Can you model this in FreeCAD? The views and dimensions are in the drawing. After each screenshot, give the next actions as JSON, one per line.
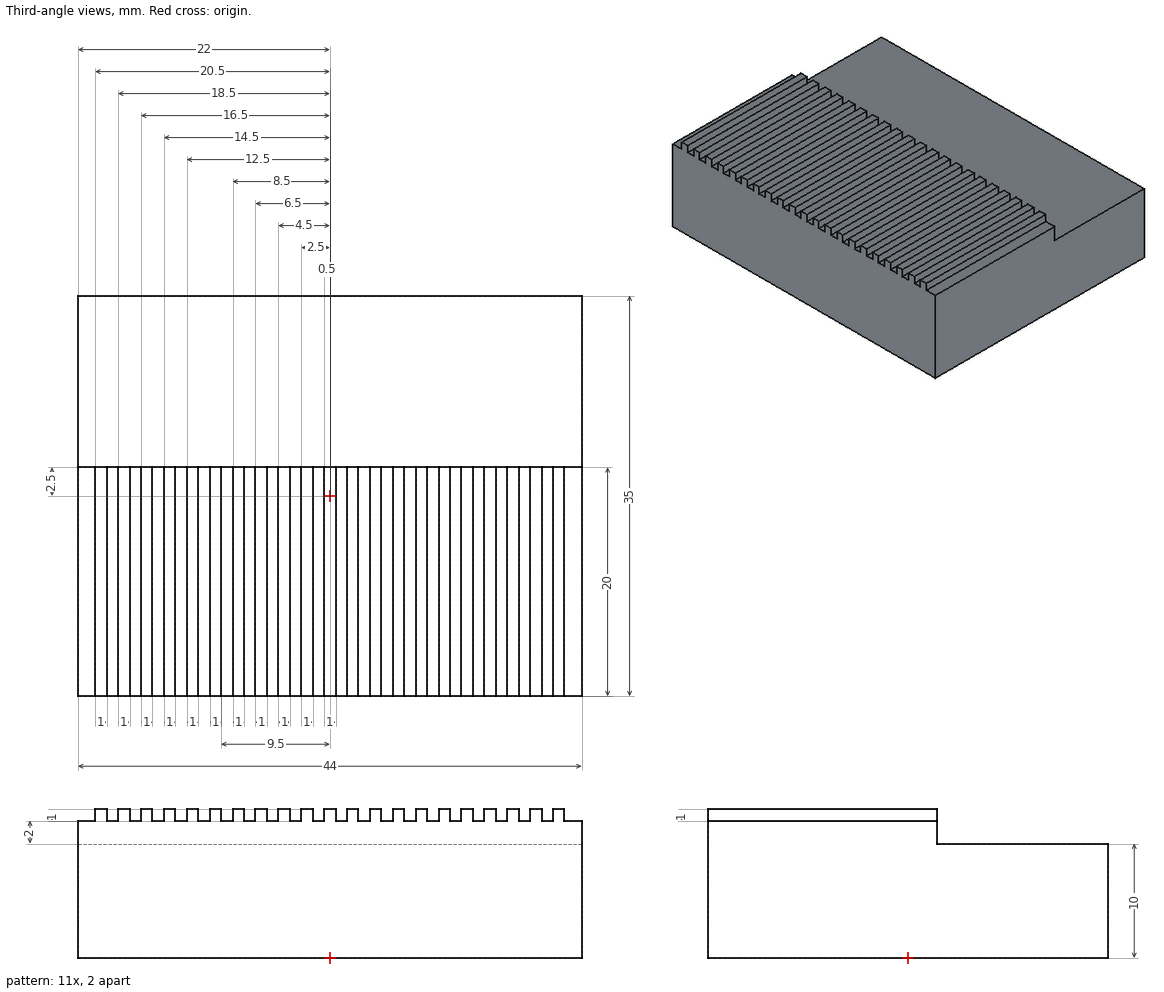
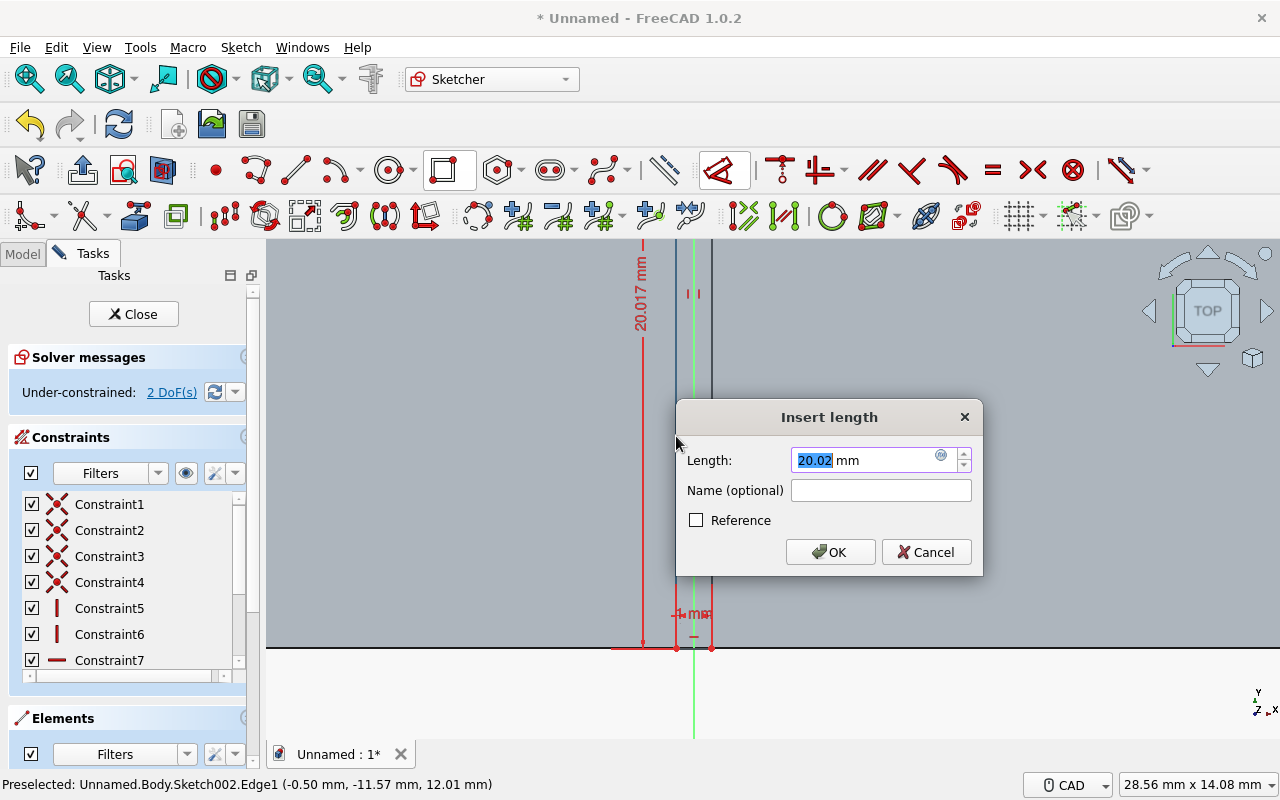
{"action": "type", "text": "20"}
{"action": "key", "text": "Return"}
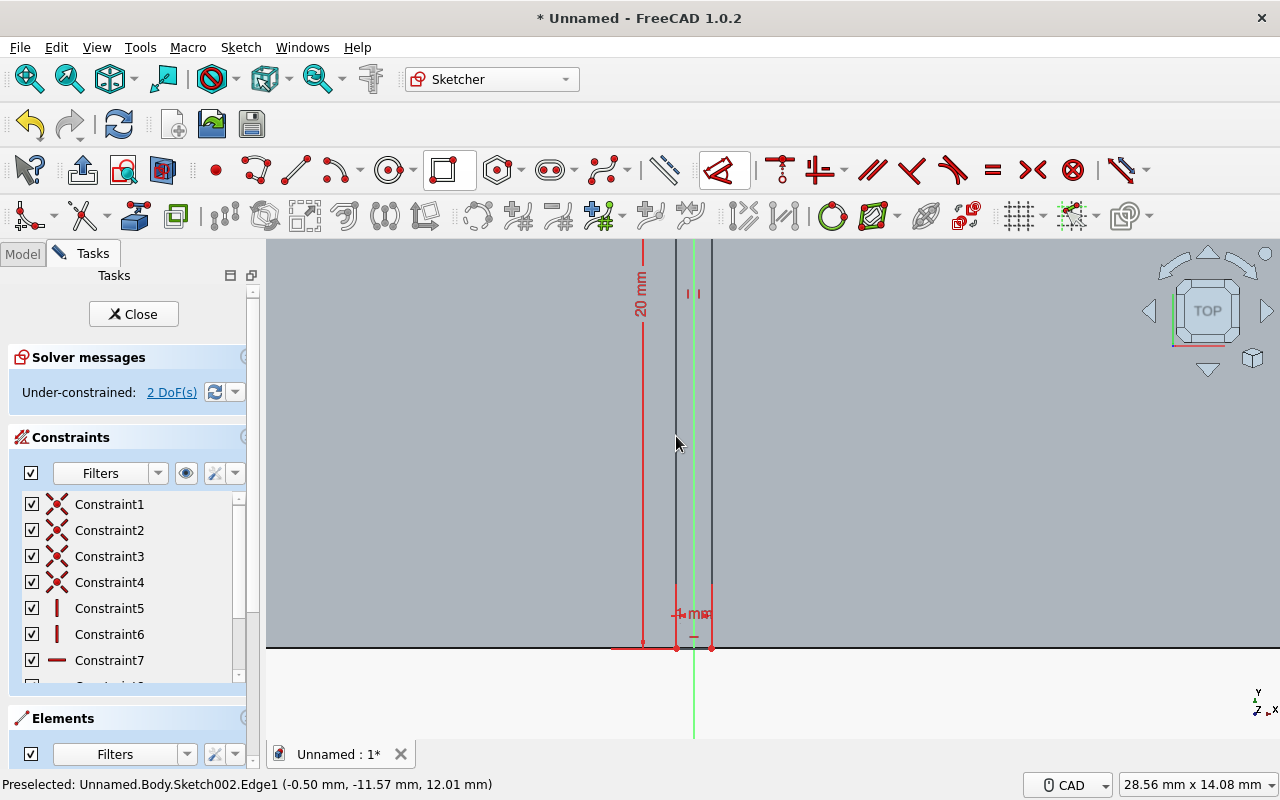
{"action": "scroll", "coordinate": [713, 649], "scroll_direction": "down", "scroll_amount": 4}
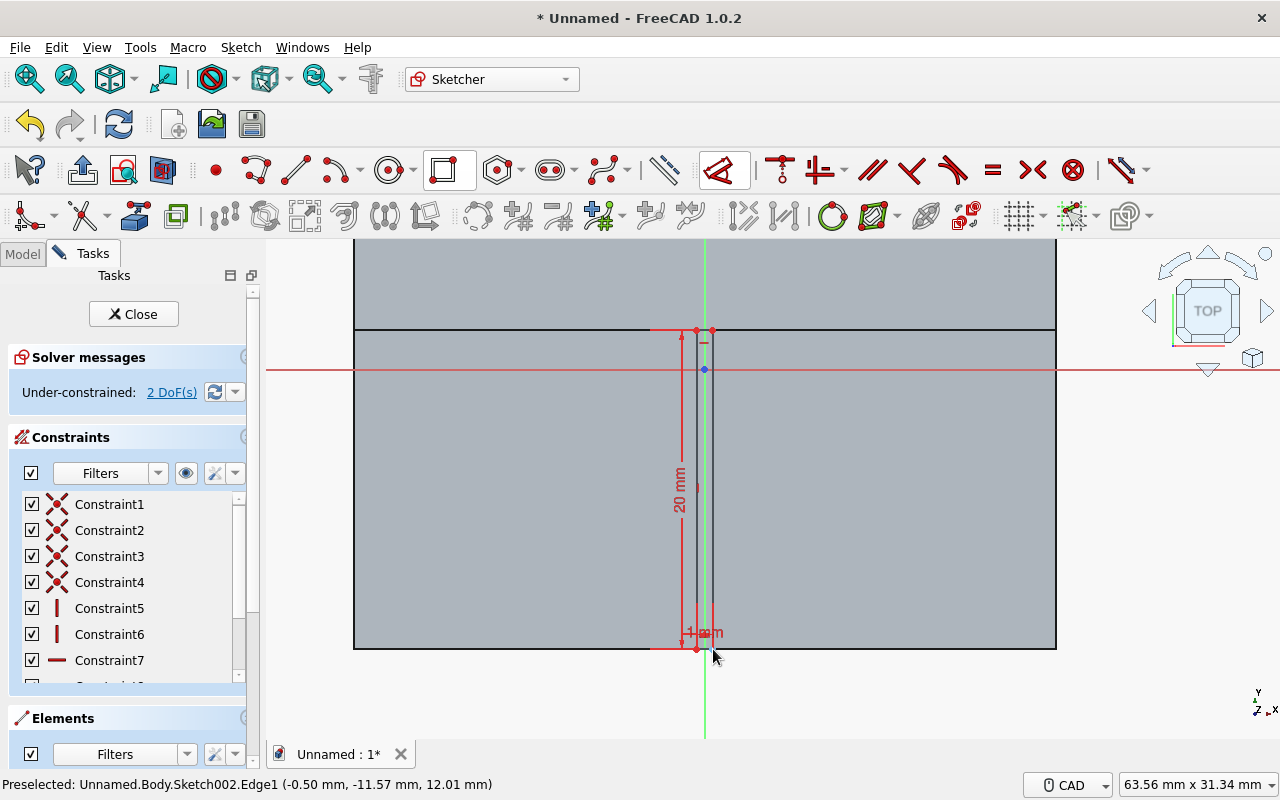
{"action": "scroll", "coordinate": [697, 330], "scroll_direction": "up", "scroll_amount": 9}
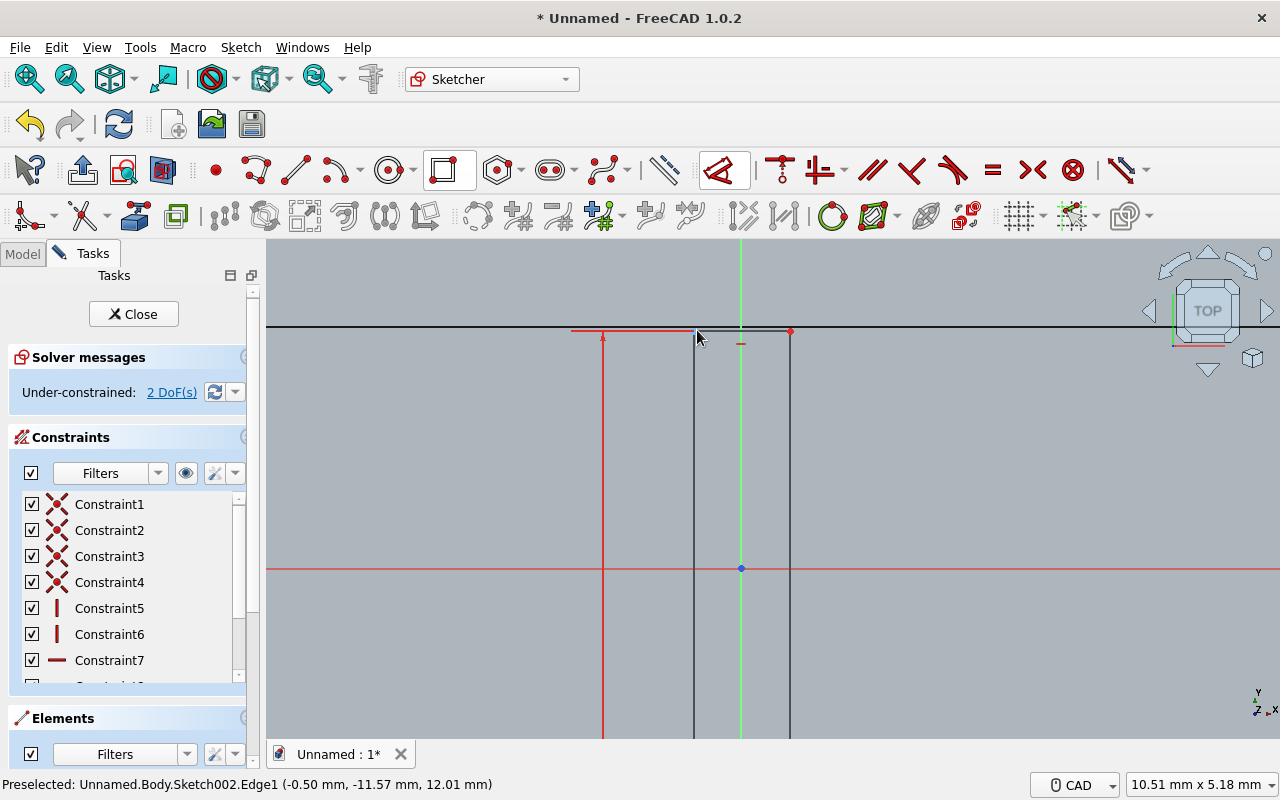
{"action": "left_click", "coordinate": [694, 331]}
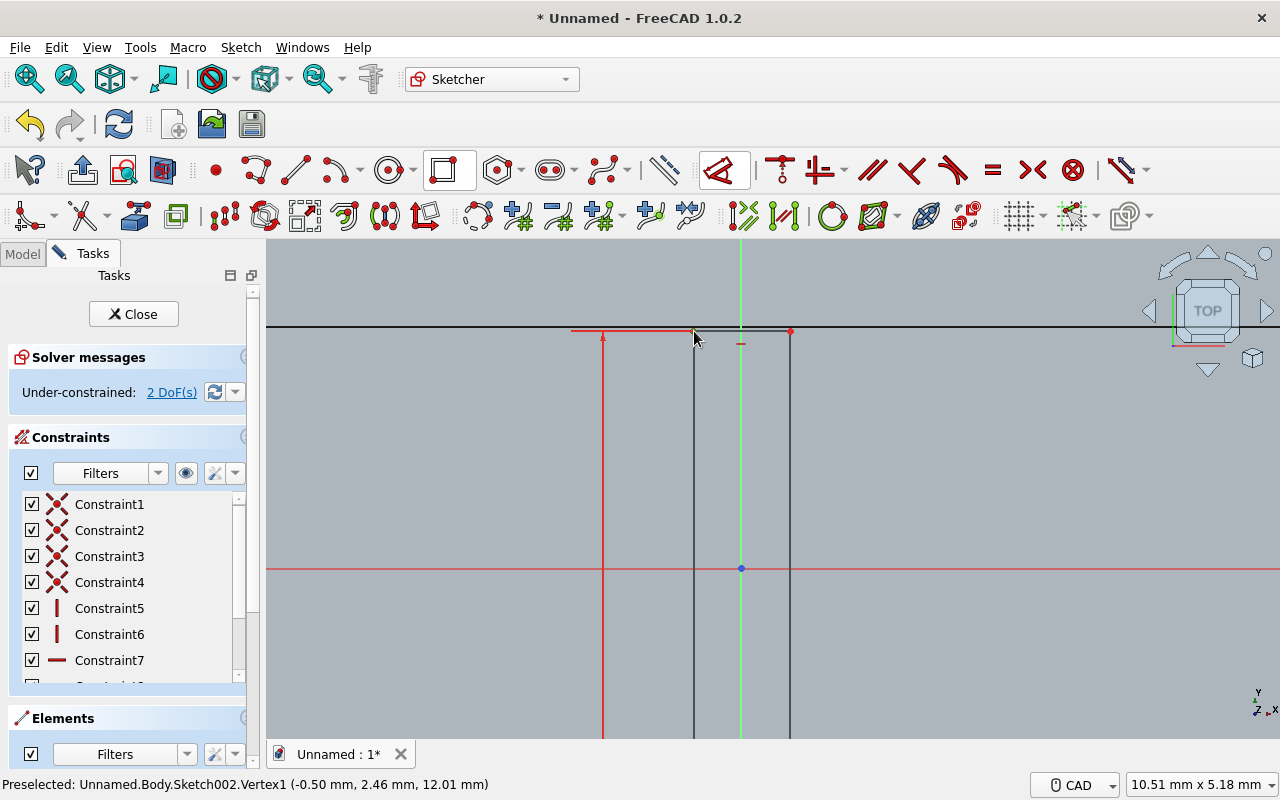
{"action": "key", "text": "l"}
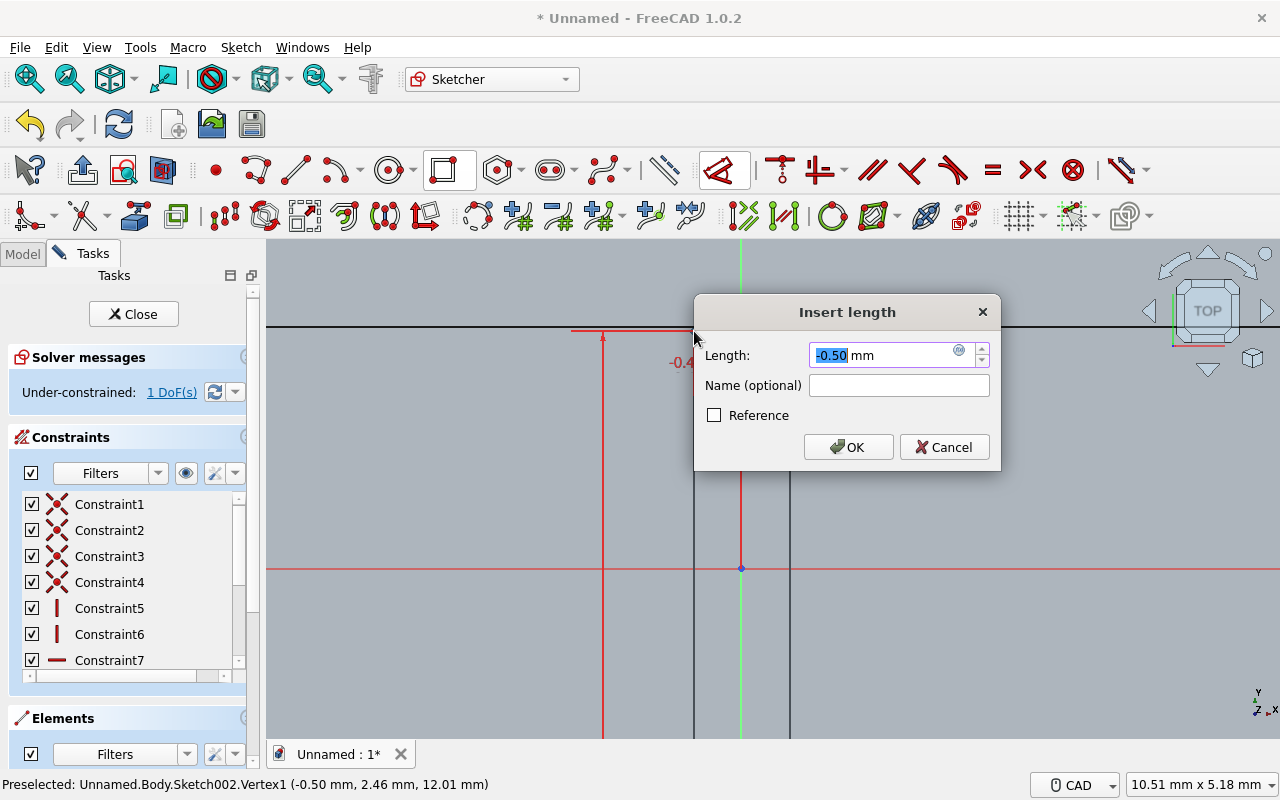
{"action": "type", "text": "-0.5"}
{"action": "key", "text": "Return"}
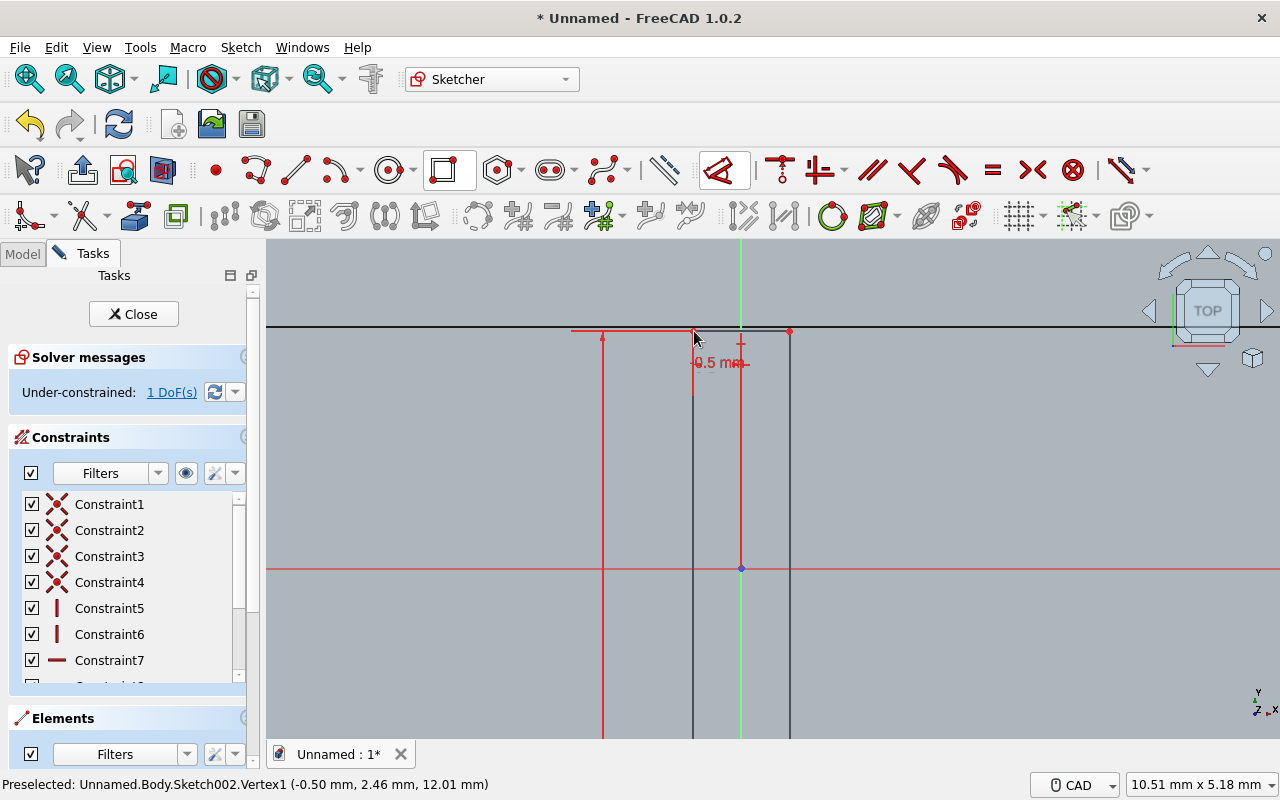
{"action": "scroll", "coordinate": [697, 330], "scroll_direction": "down", "scroll_amount": 9}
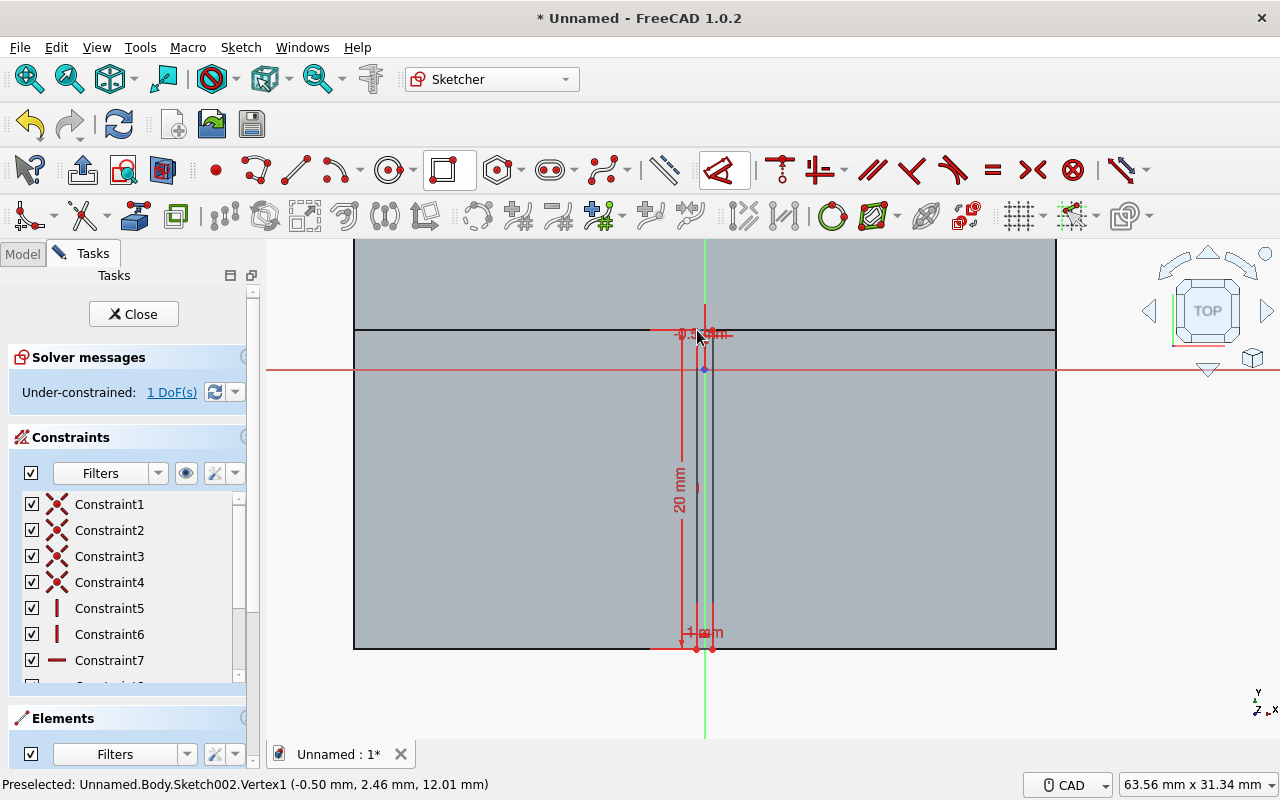
{"action": "left_click", "coordinate": [697, 330]}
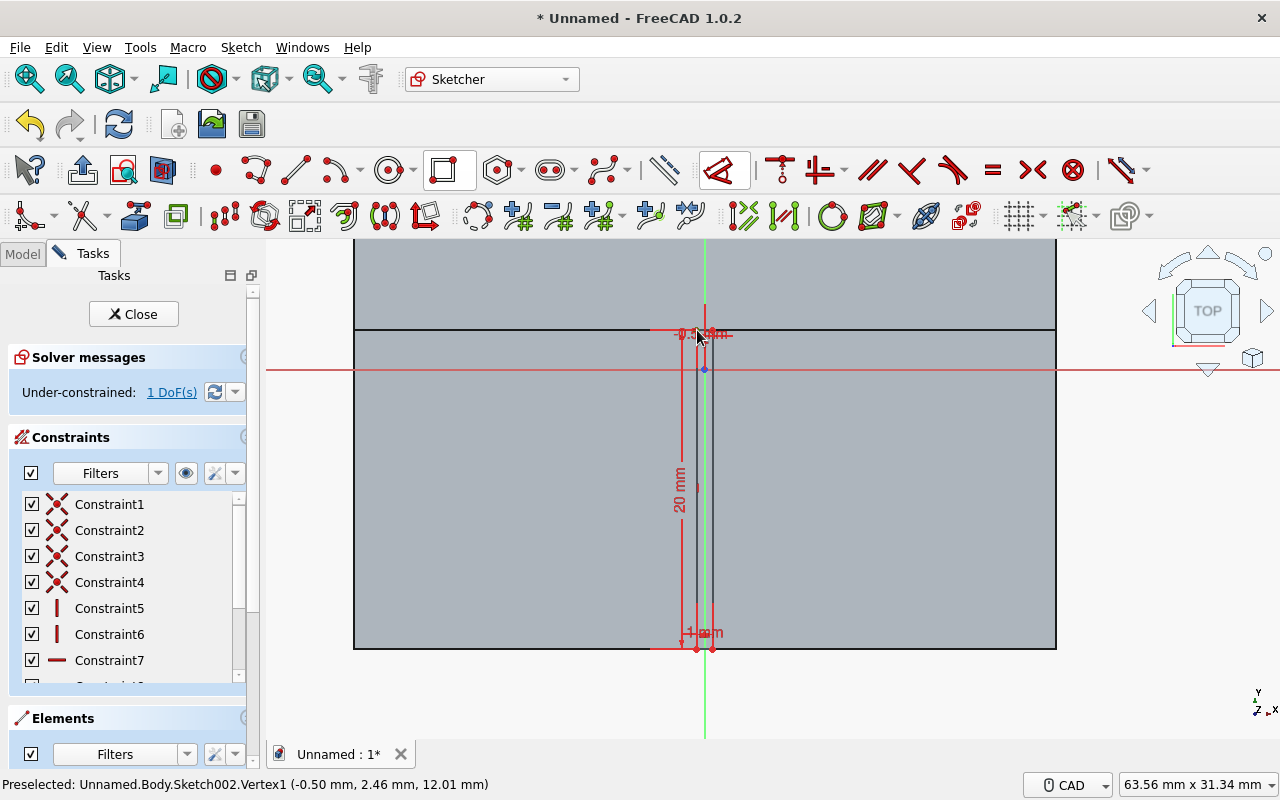
{"action": "left_click", "coordinate": [744, 170]}